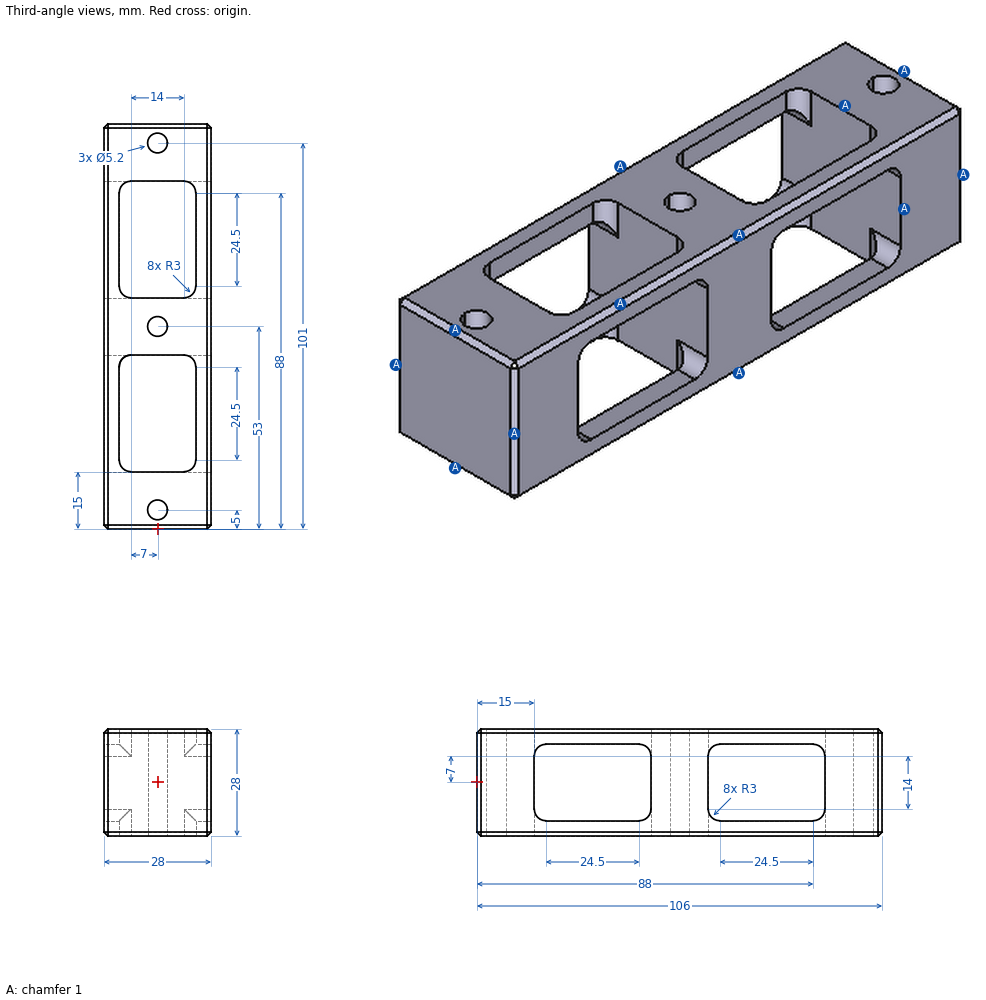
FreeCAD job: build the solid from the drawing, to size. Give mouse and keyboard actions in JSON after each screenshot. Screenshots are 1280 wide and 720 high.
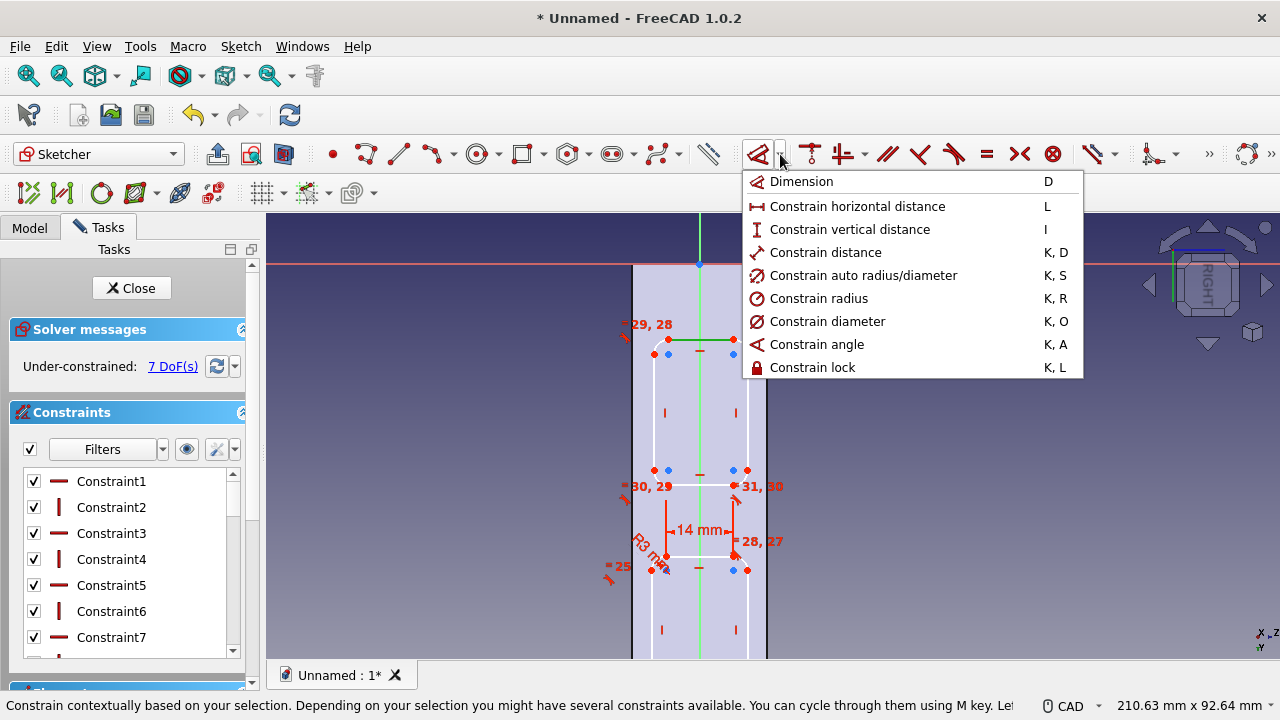
{"action": "left_click", "coordinate": [913, 206]}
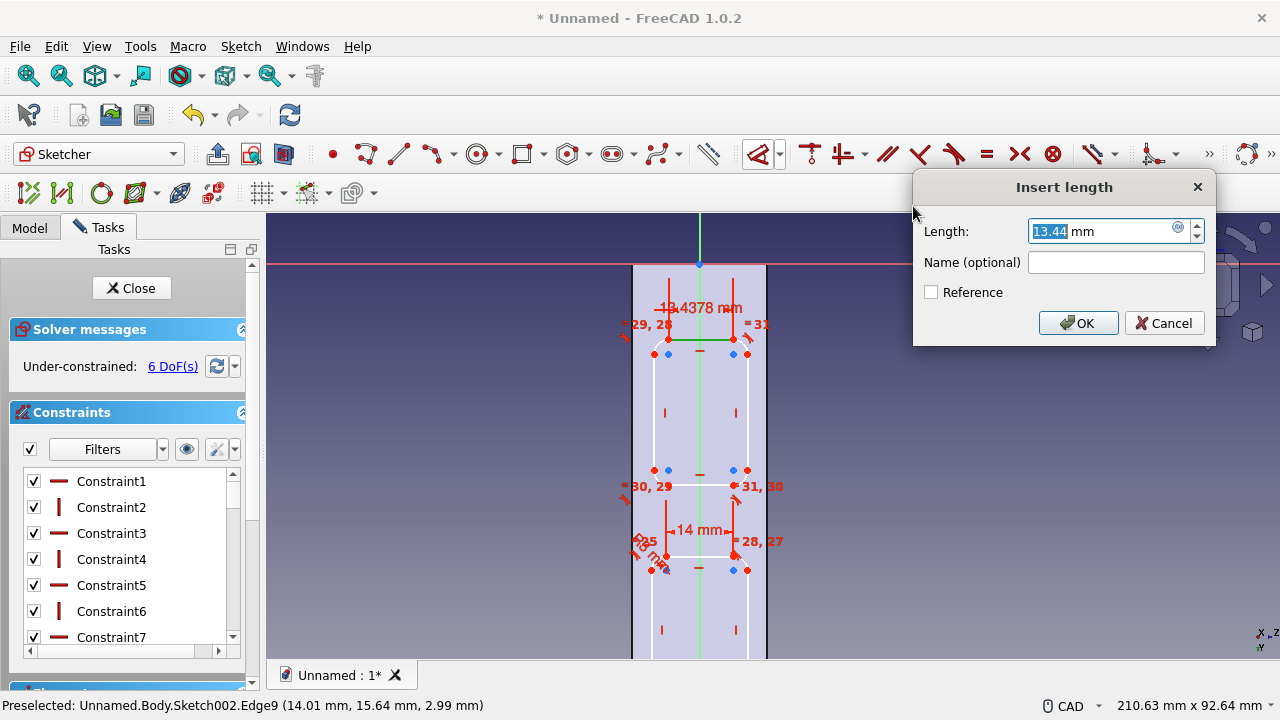
{"action": "type", "text": "14"}
{"action": "key", "text": "Return"}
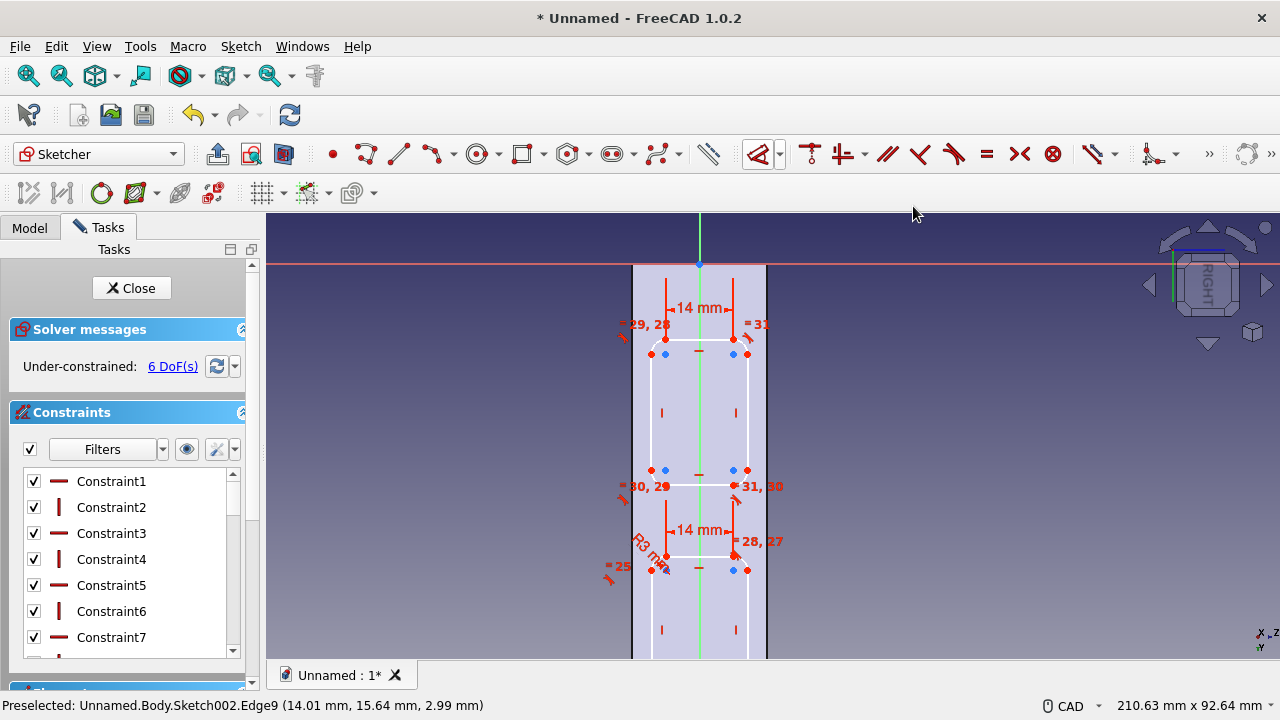
{"action": "left_click", "coordinate": [733, 557]}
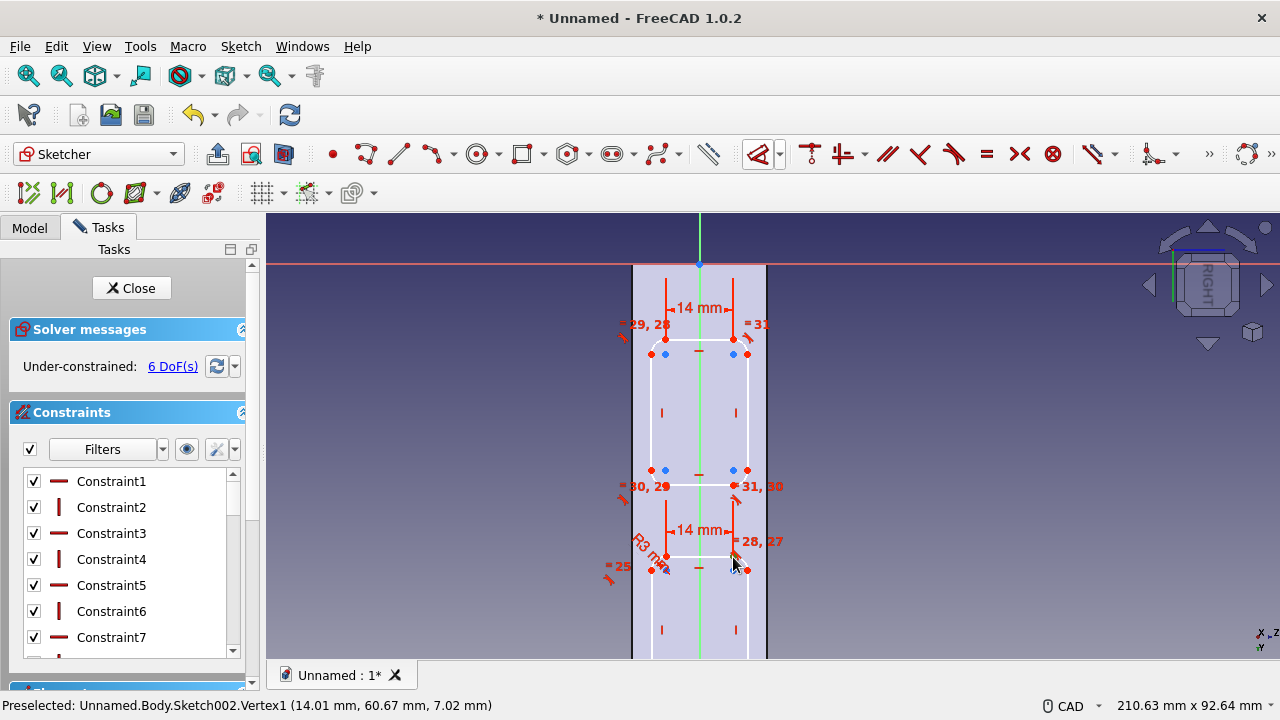
{"action": "left_click", "coordinate": [780, 154]}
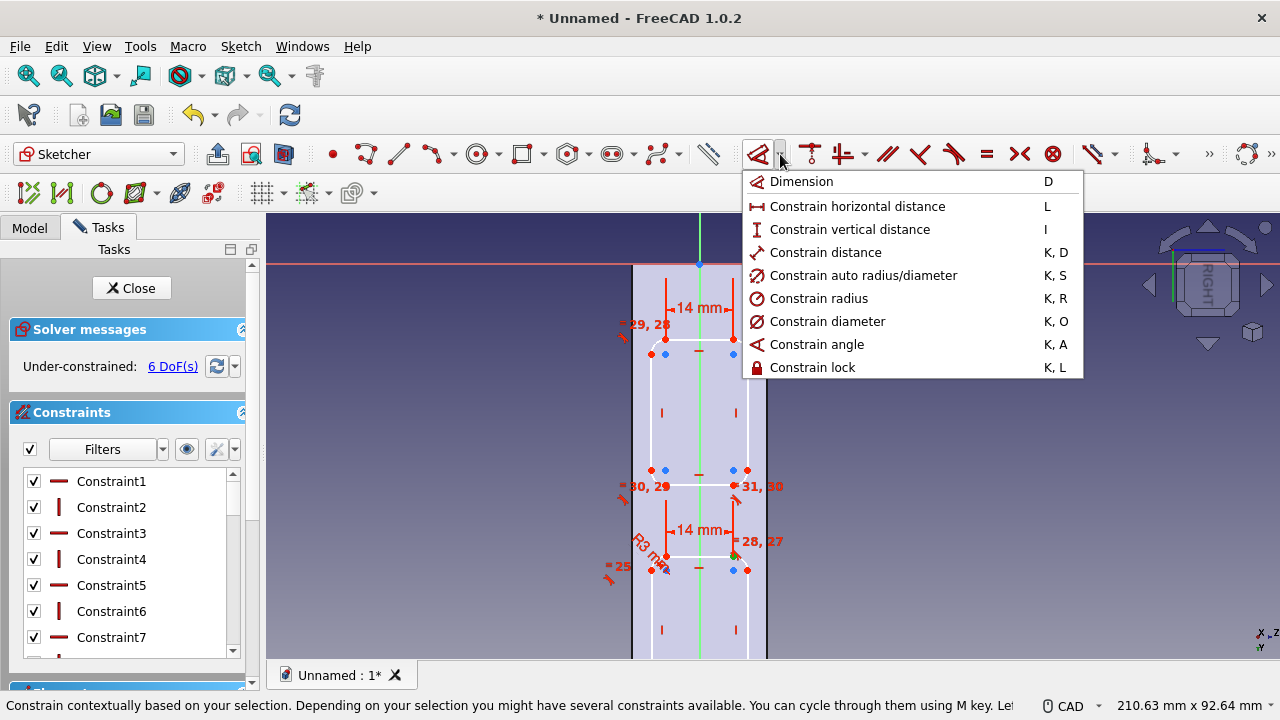
{"action": "left_click", "coordinate": [913, 206]}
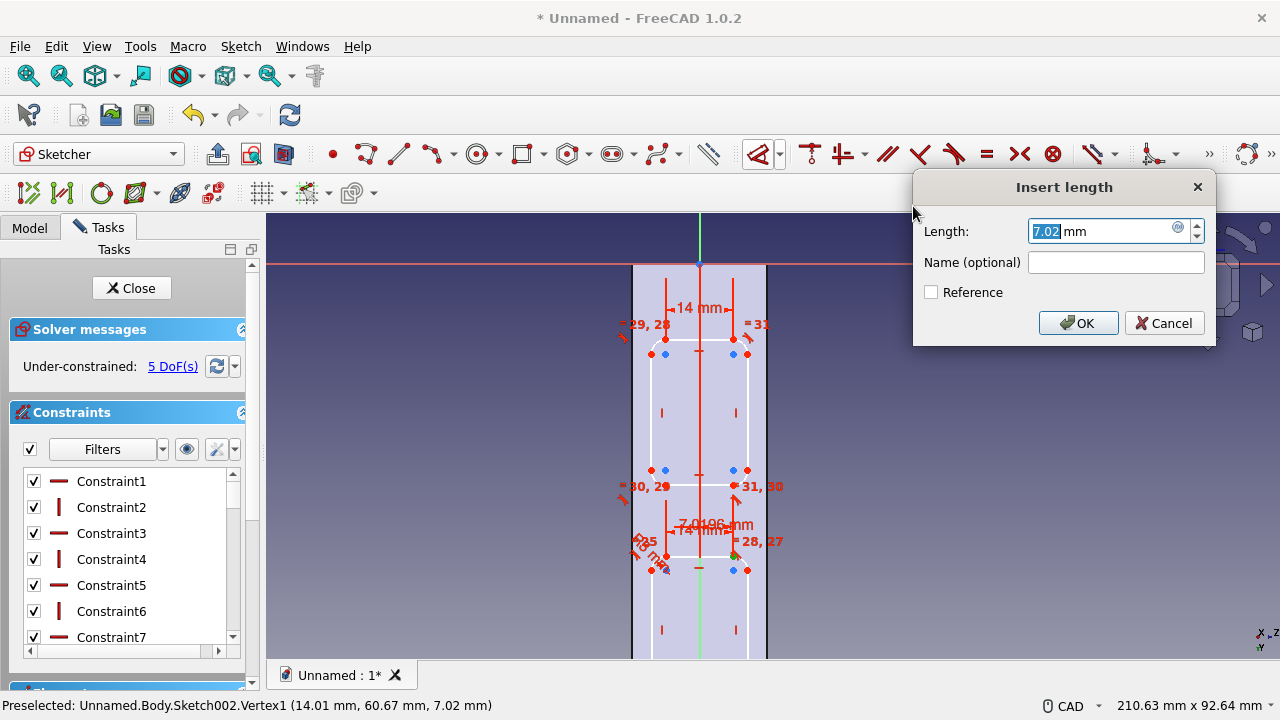
{"action": "type", "text": "7"}
{"action": "key", "text": "Return"}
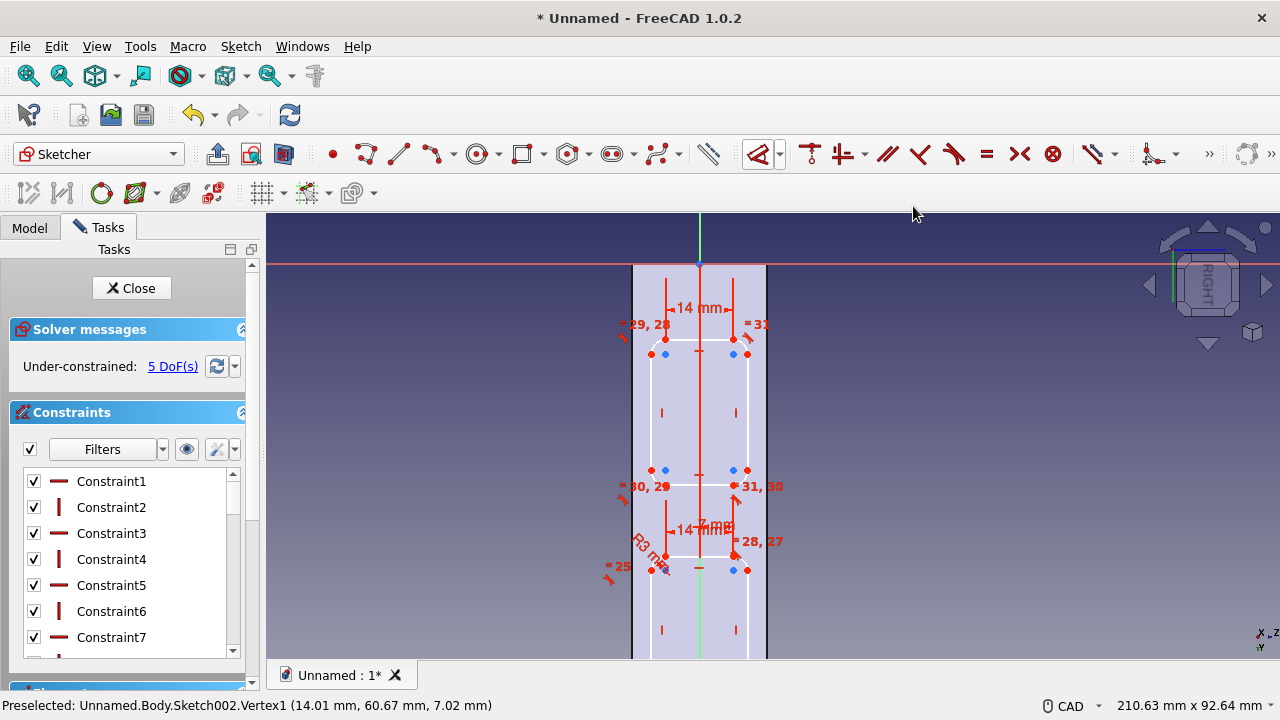
{"action": "left_click", "coordinate": [733, 340]}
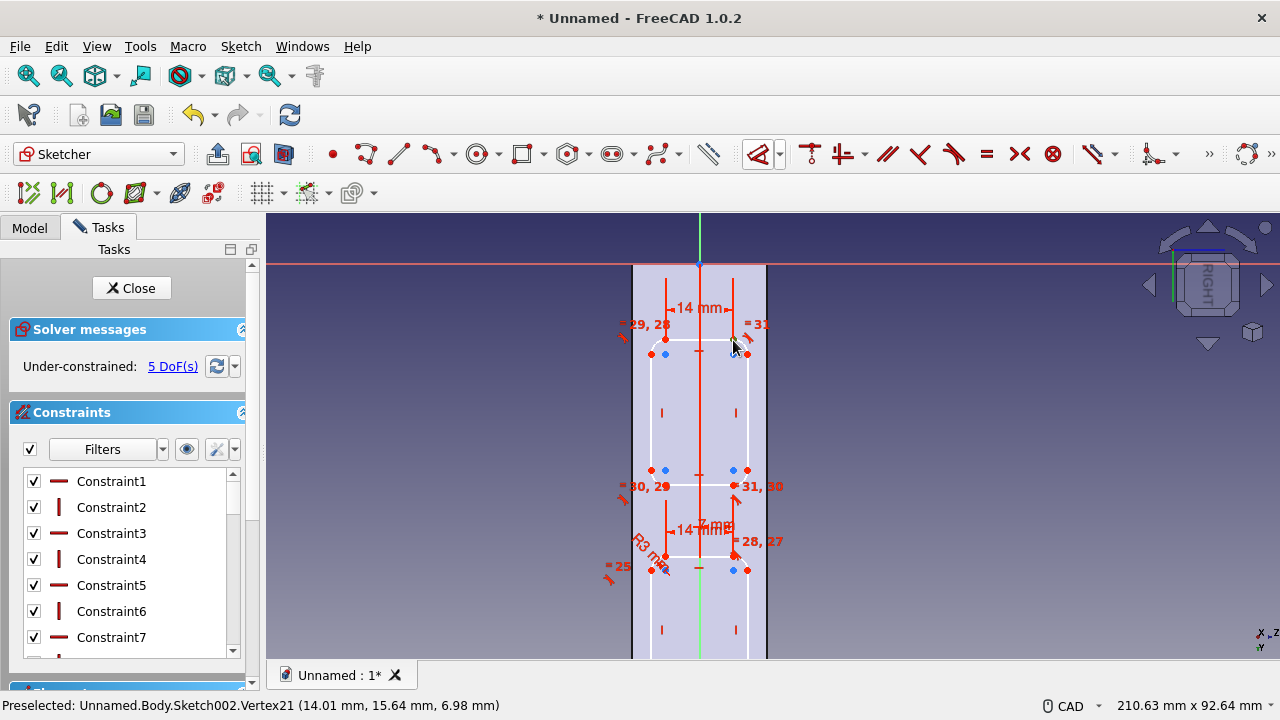
{"action": "left_click", "coordinate": [780, 154]}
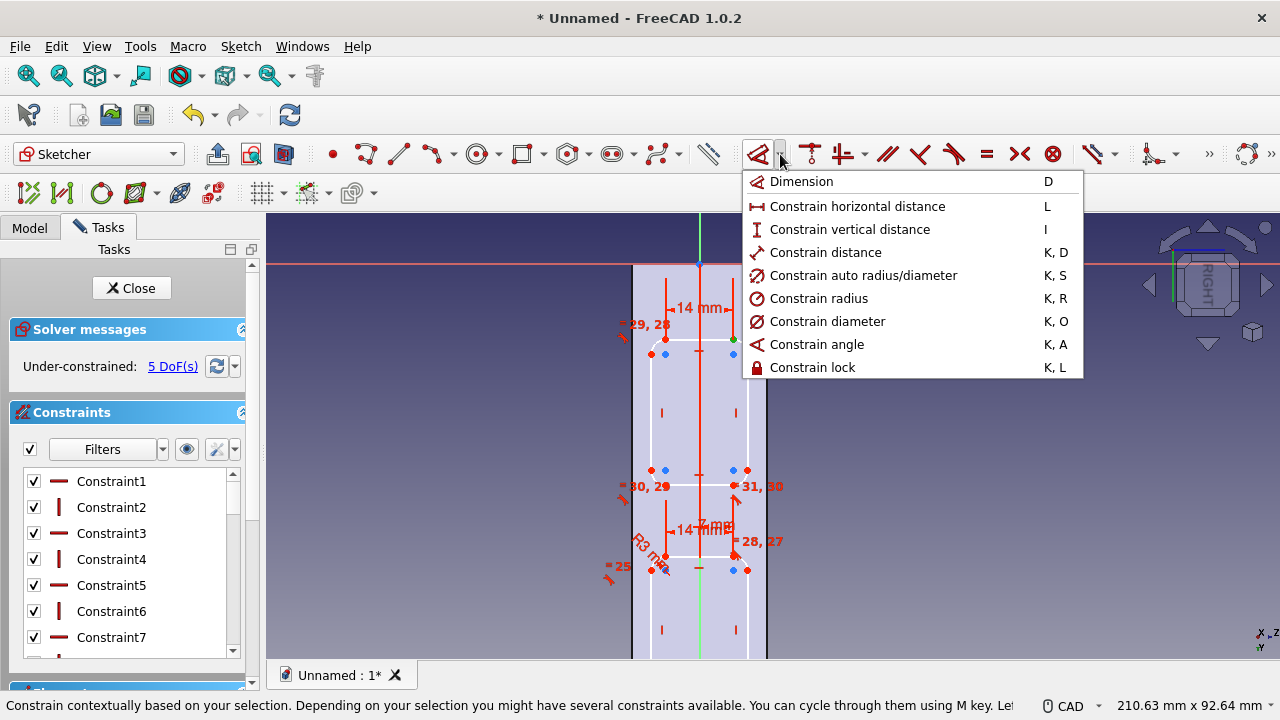
{"action": "left_click", "coordinate": [913, 206]}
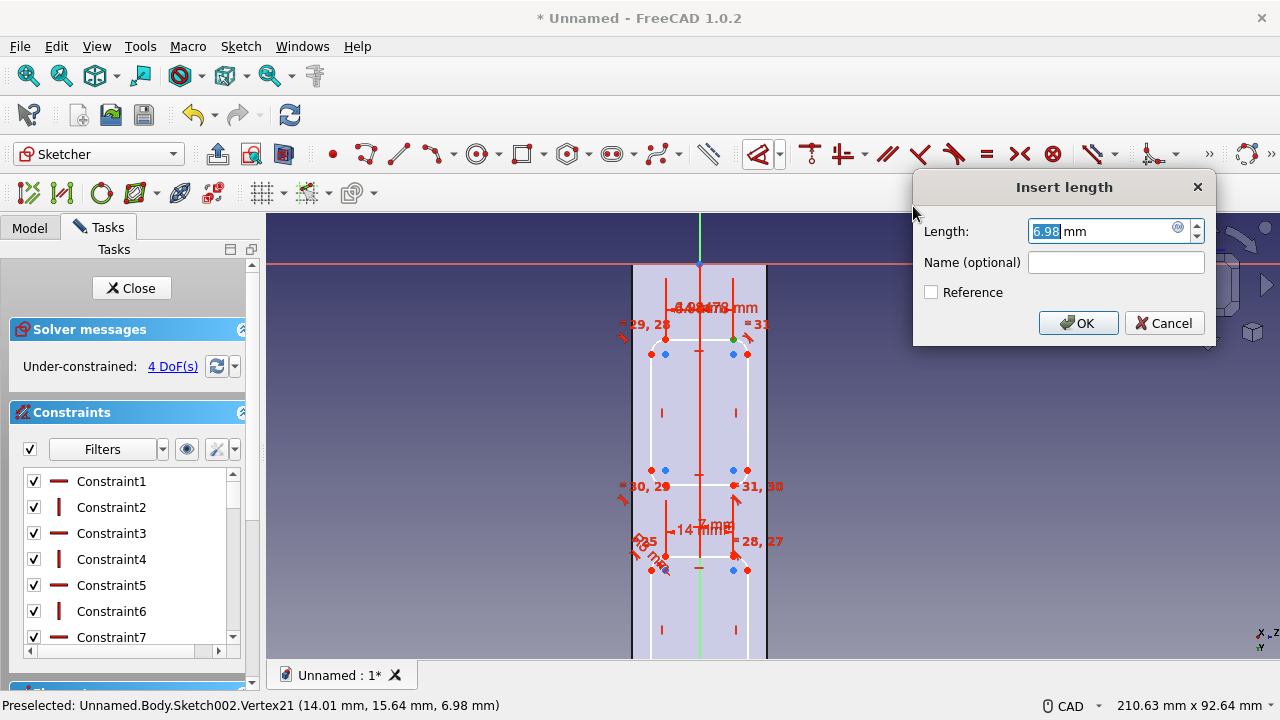
{"action": "type", "text": "7"}
{"action": "key", "text": "Return"}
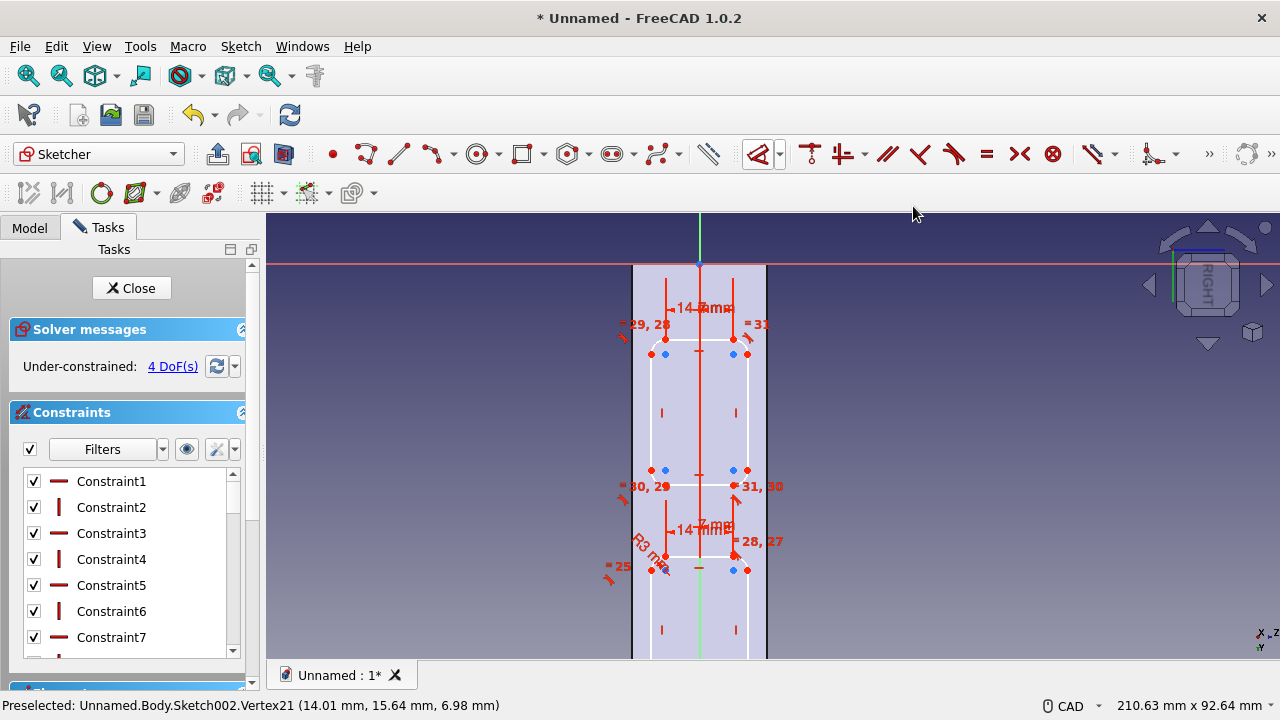
{"action": "scroll", "coordinate": [714, 339], "scroll_direction": "down", "scroll_amount": 2}